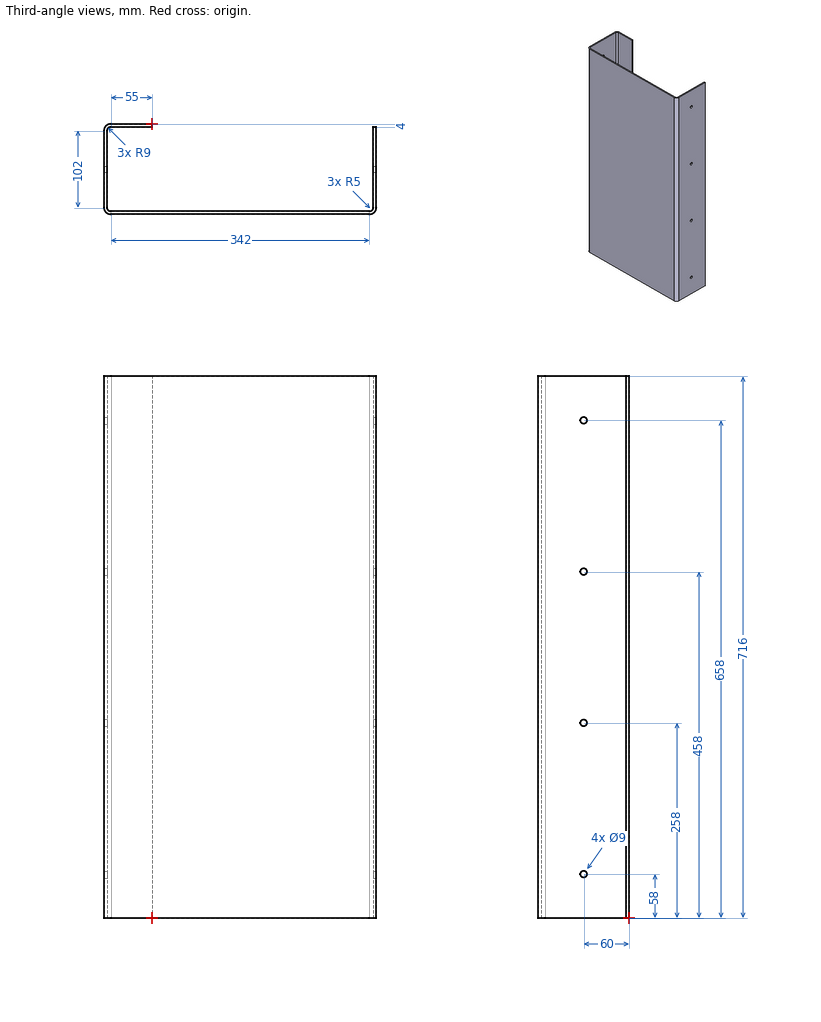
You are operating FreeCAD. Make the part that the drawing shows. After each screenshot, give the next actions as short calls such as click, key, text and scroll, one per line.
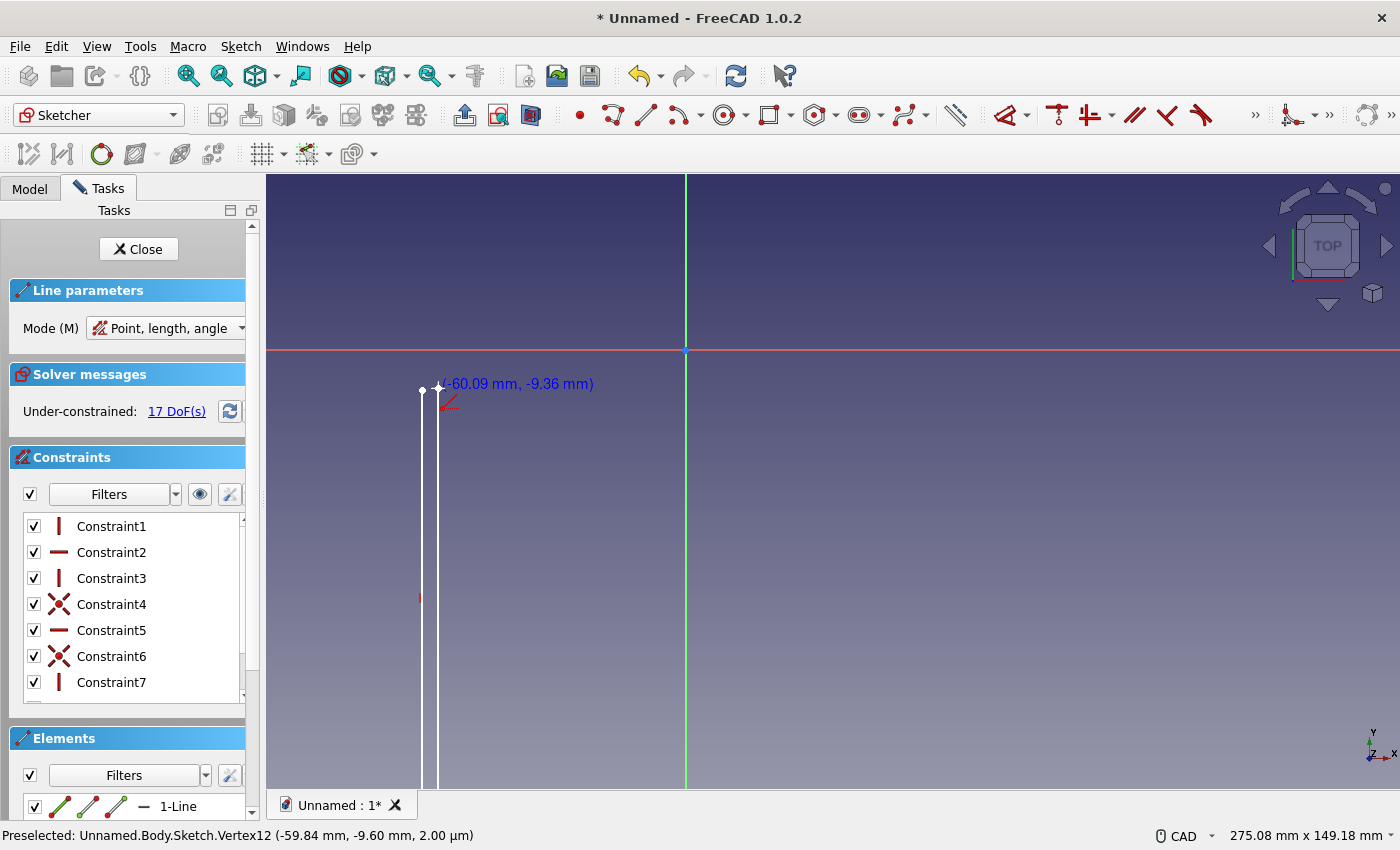
click(613, 116)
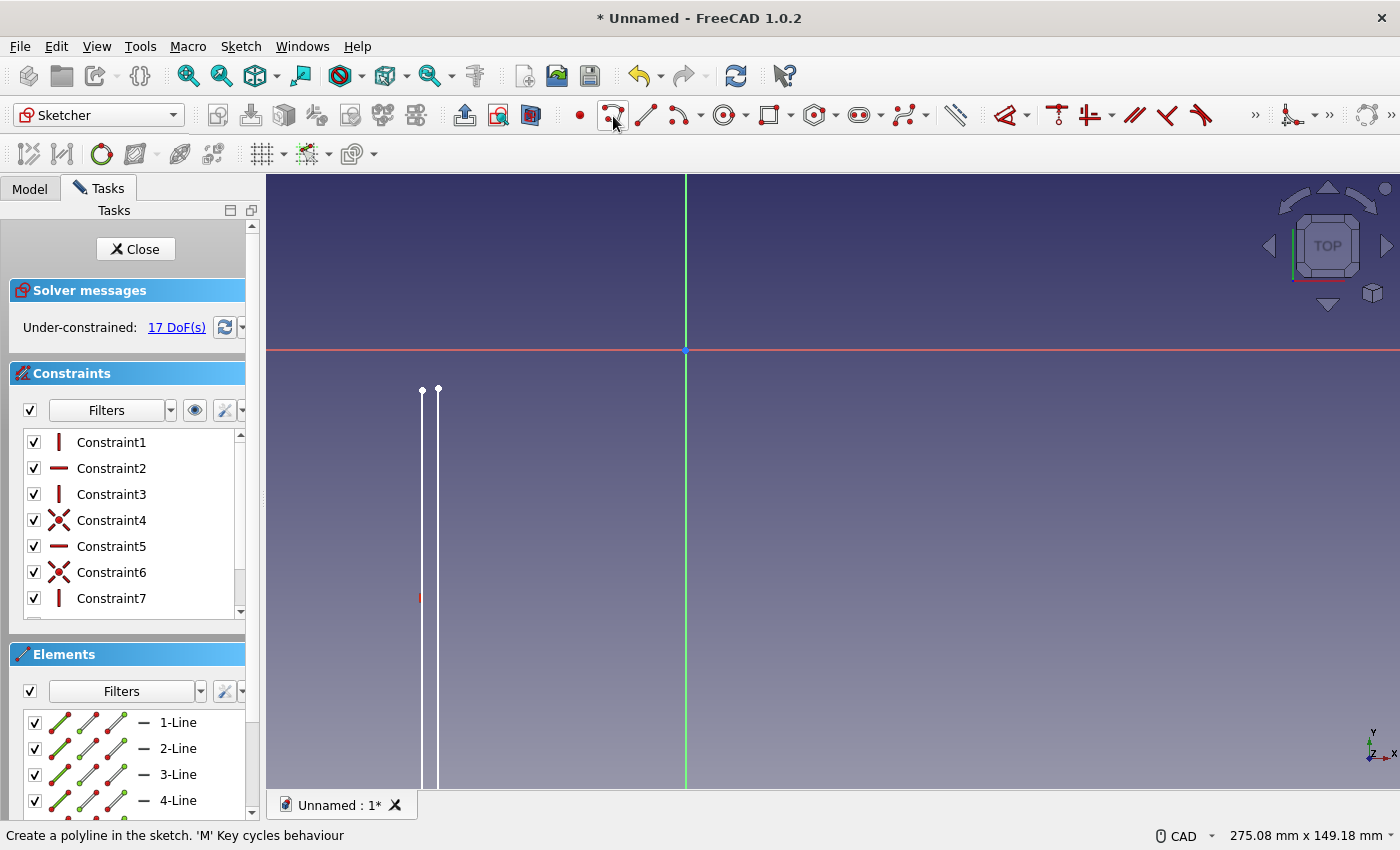
click(459, 367)
click(686, 367)
click(686, 350)
click(459, 359)
right_click(459, 359)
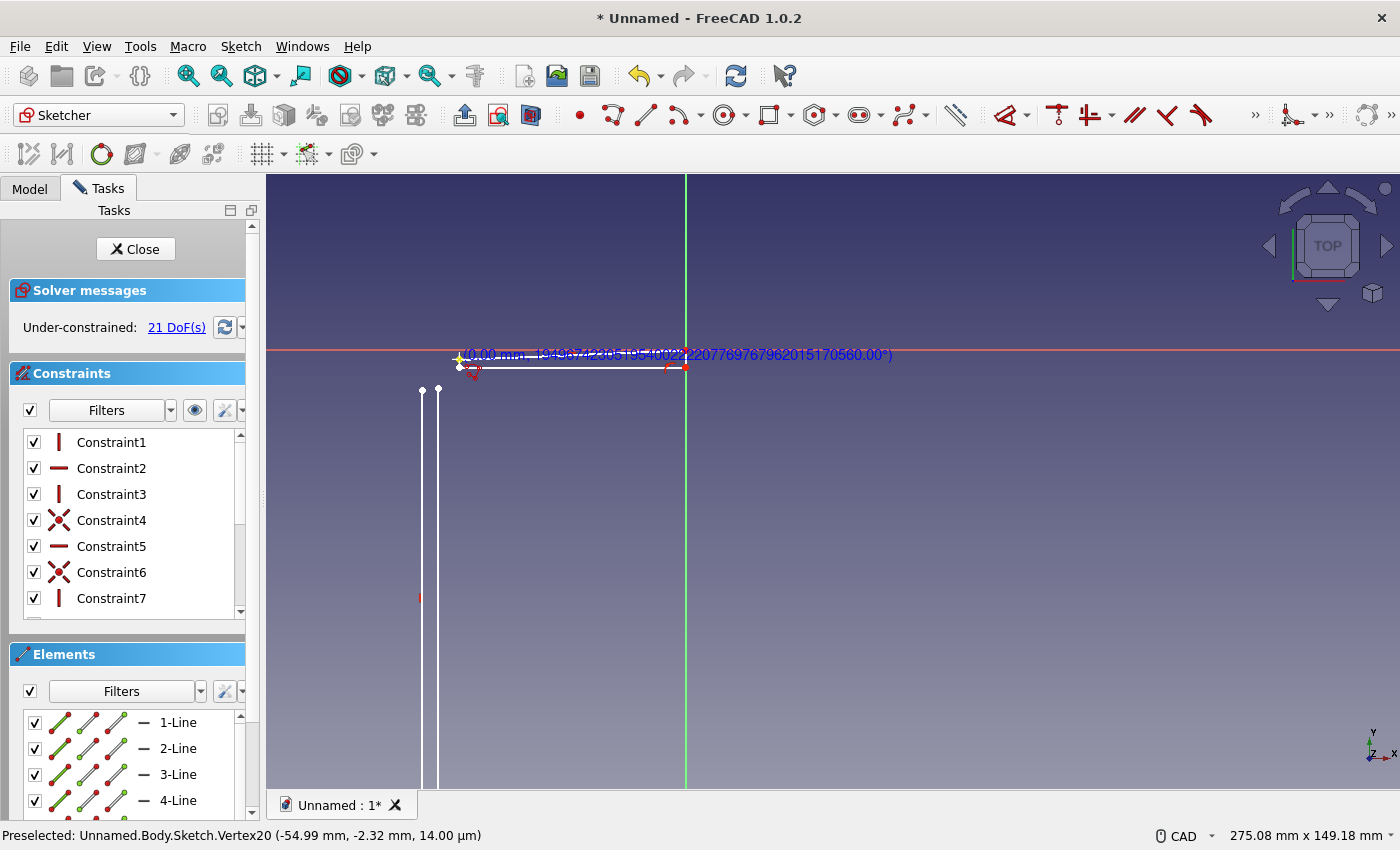
key(g)
key(3)
key(a)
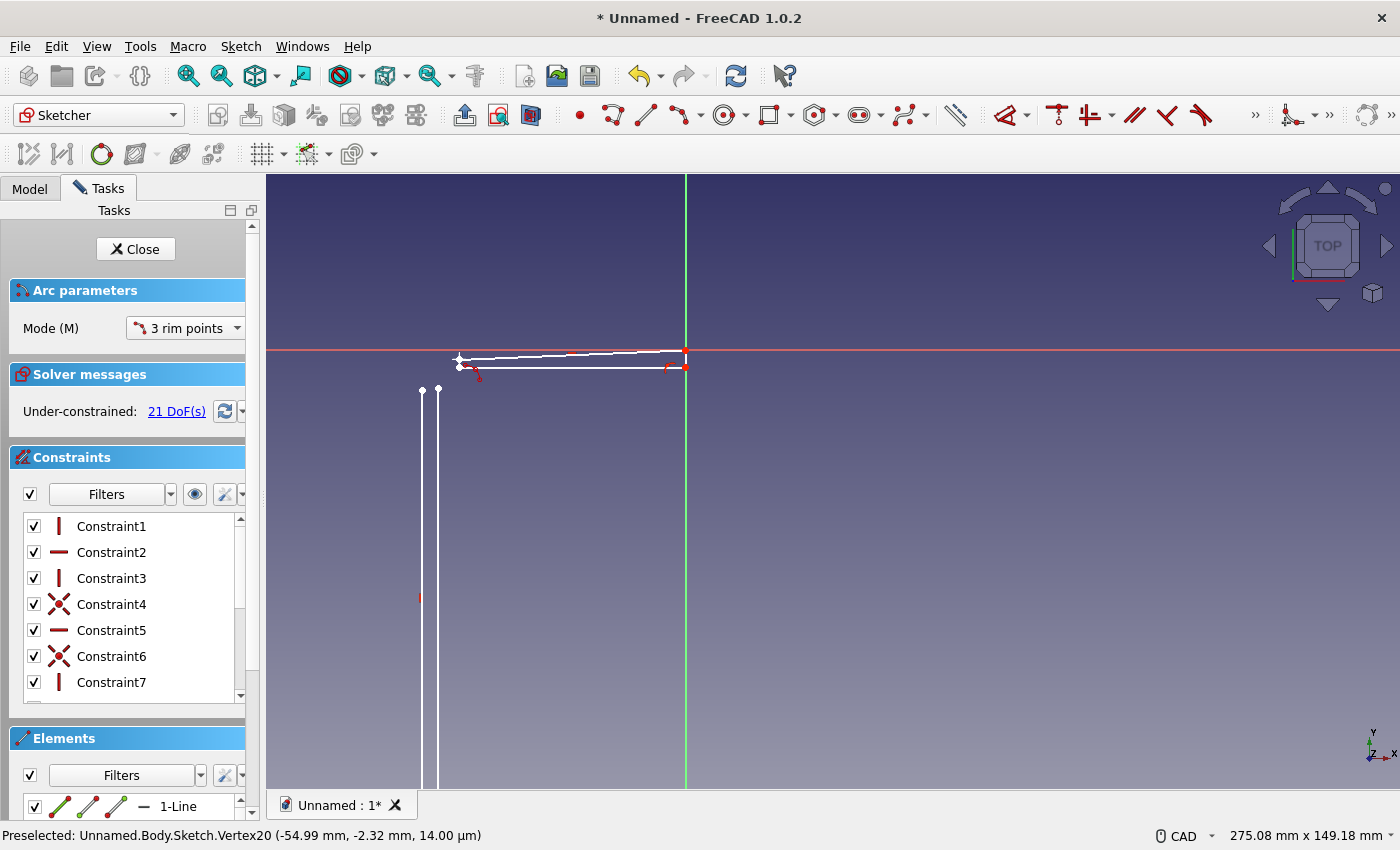
scroll(439, 387, down, 4)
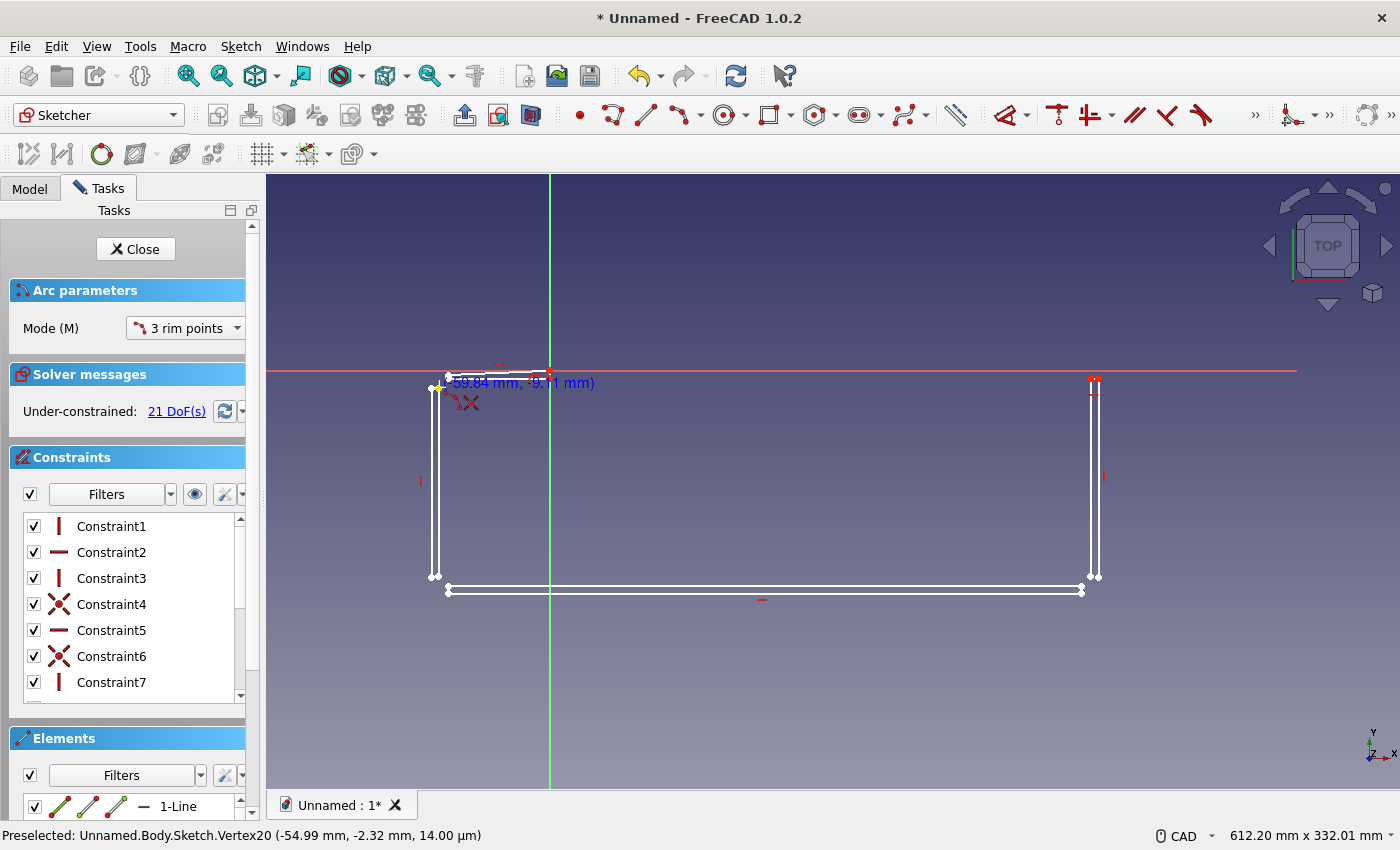
scroll(431, 576, up, 4)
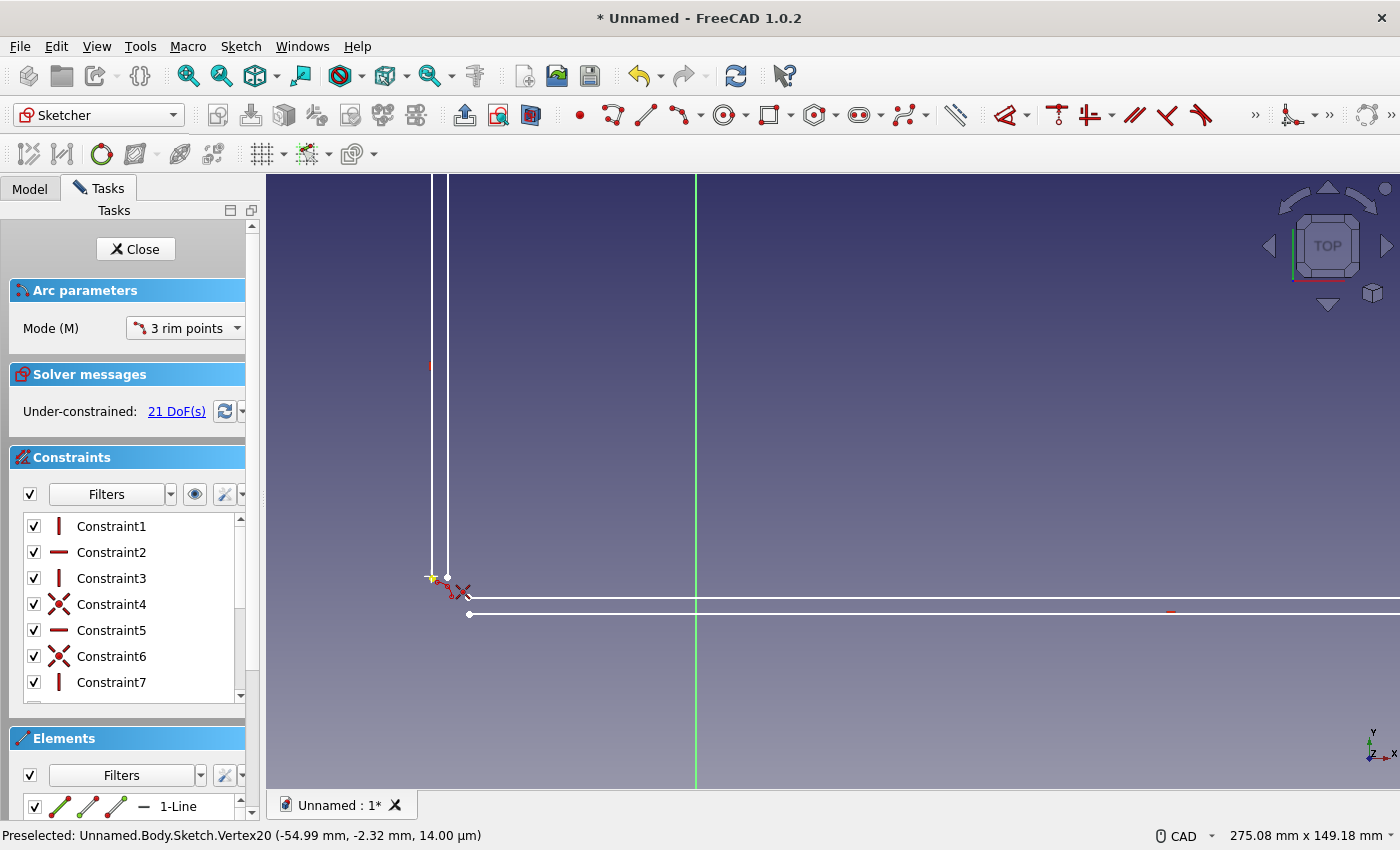
click(432, 579)
click(470, 614)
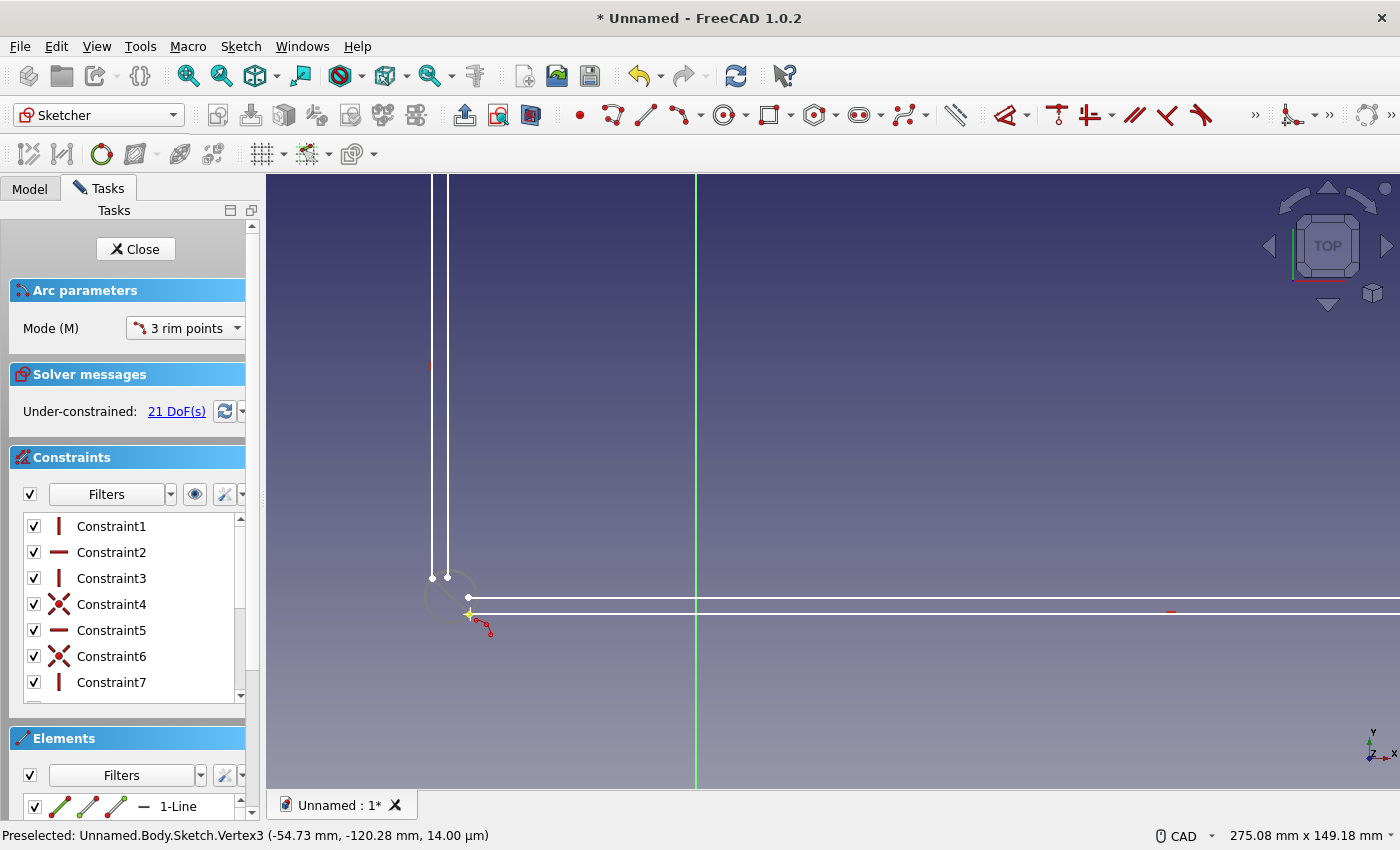
scroll(443, 602, up, 2)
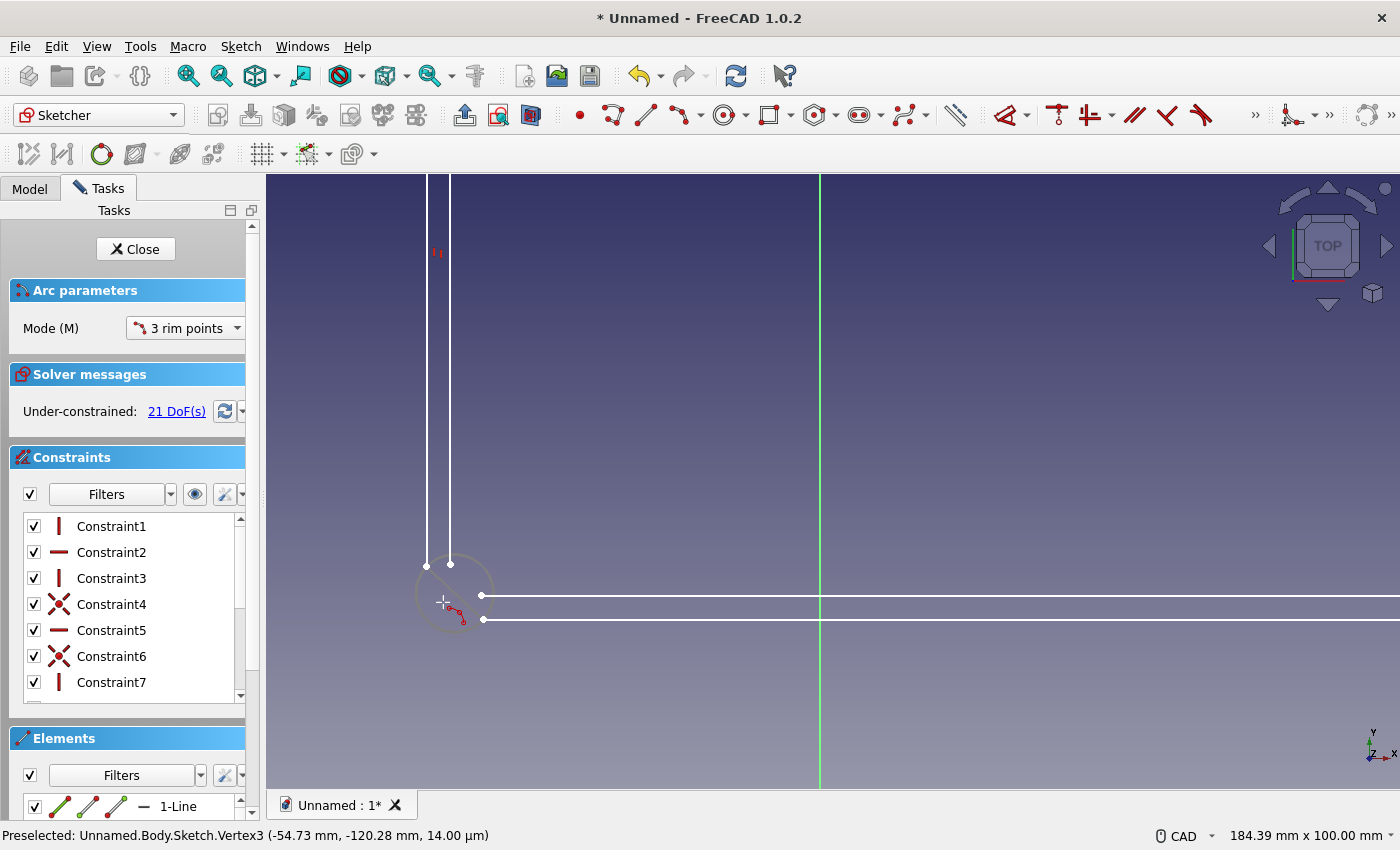
click(442, 602)